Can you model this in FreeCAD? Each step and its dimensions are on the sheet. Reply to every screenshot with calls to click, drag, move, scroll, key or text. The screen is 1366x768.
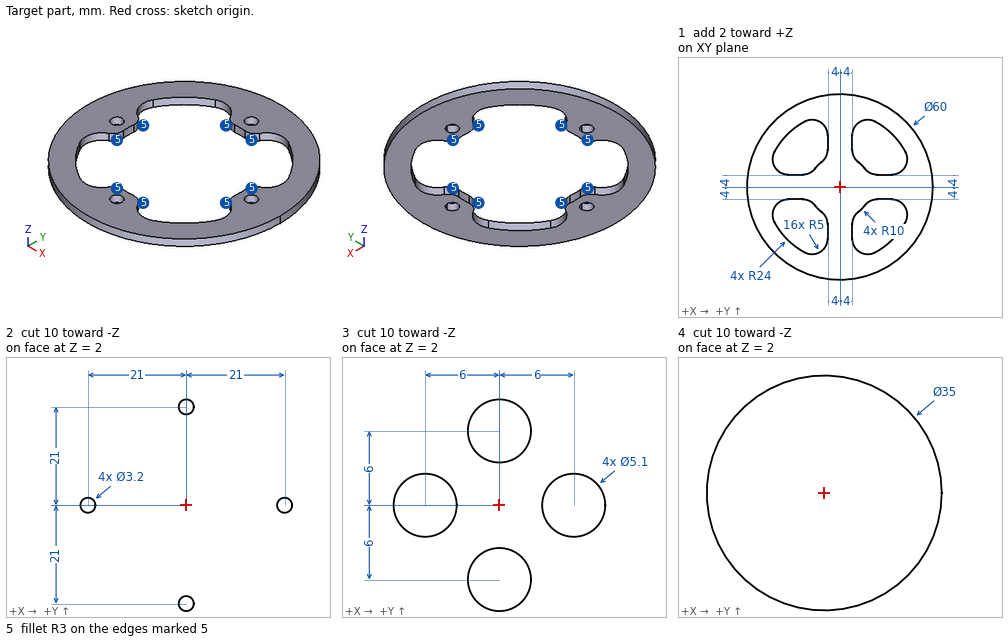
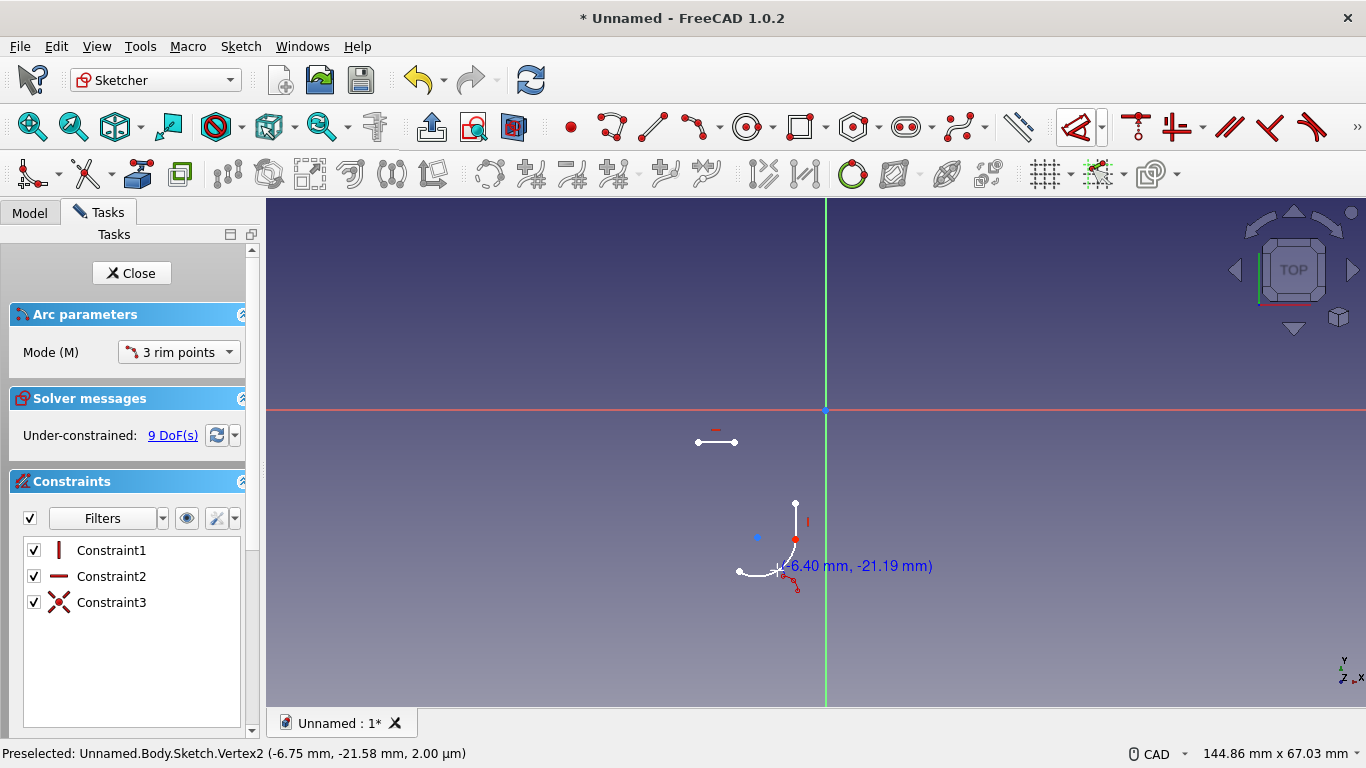
click(739, 572)
click(665, 496)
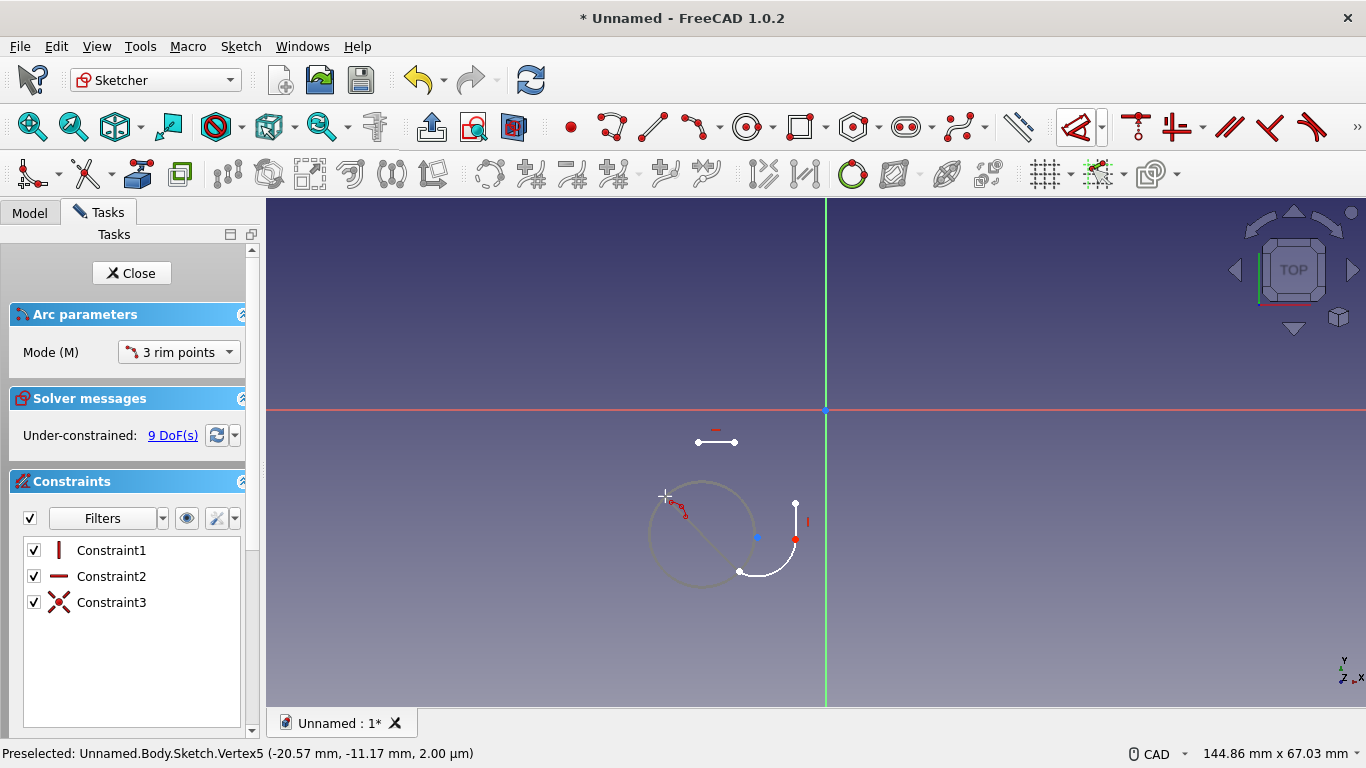
scroll(697, 539, up, 4)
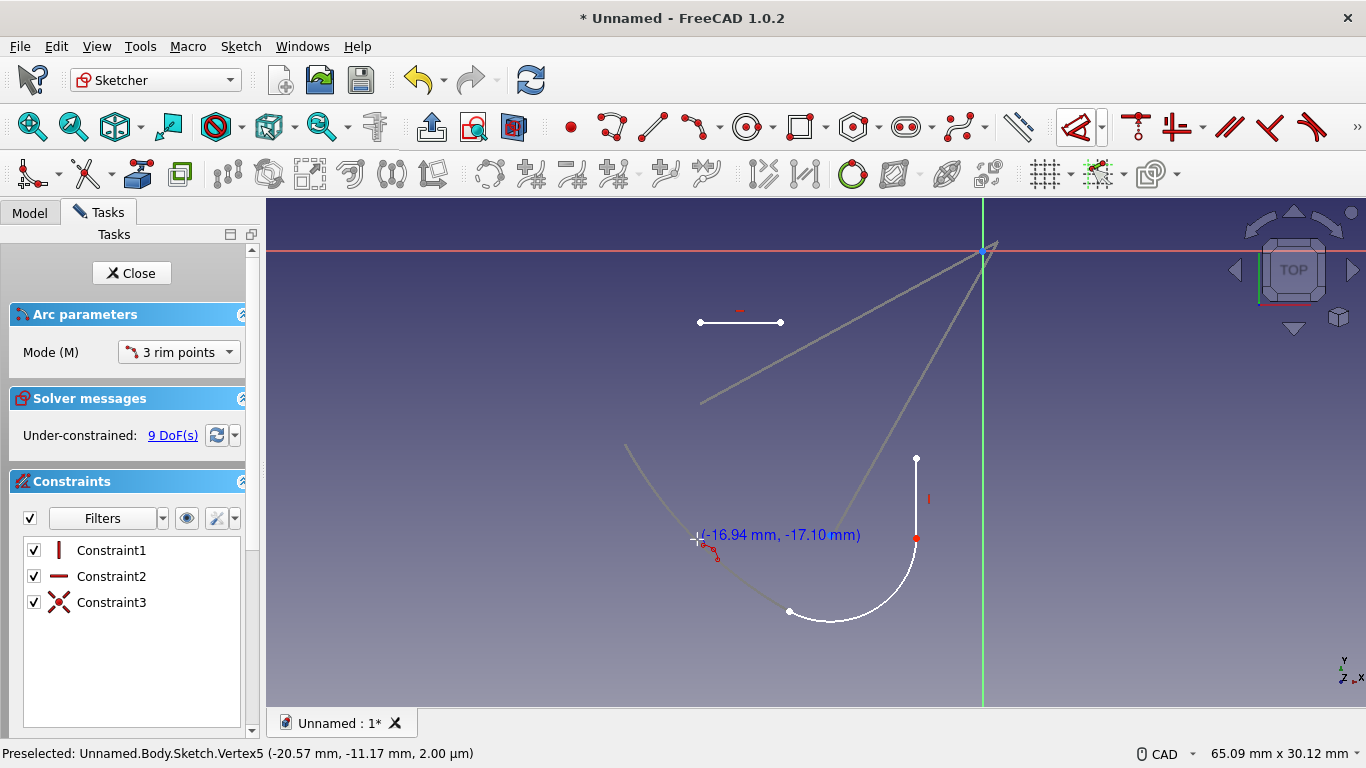
click(696, 538)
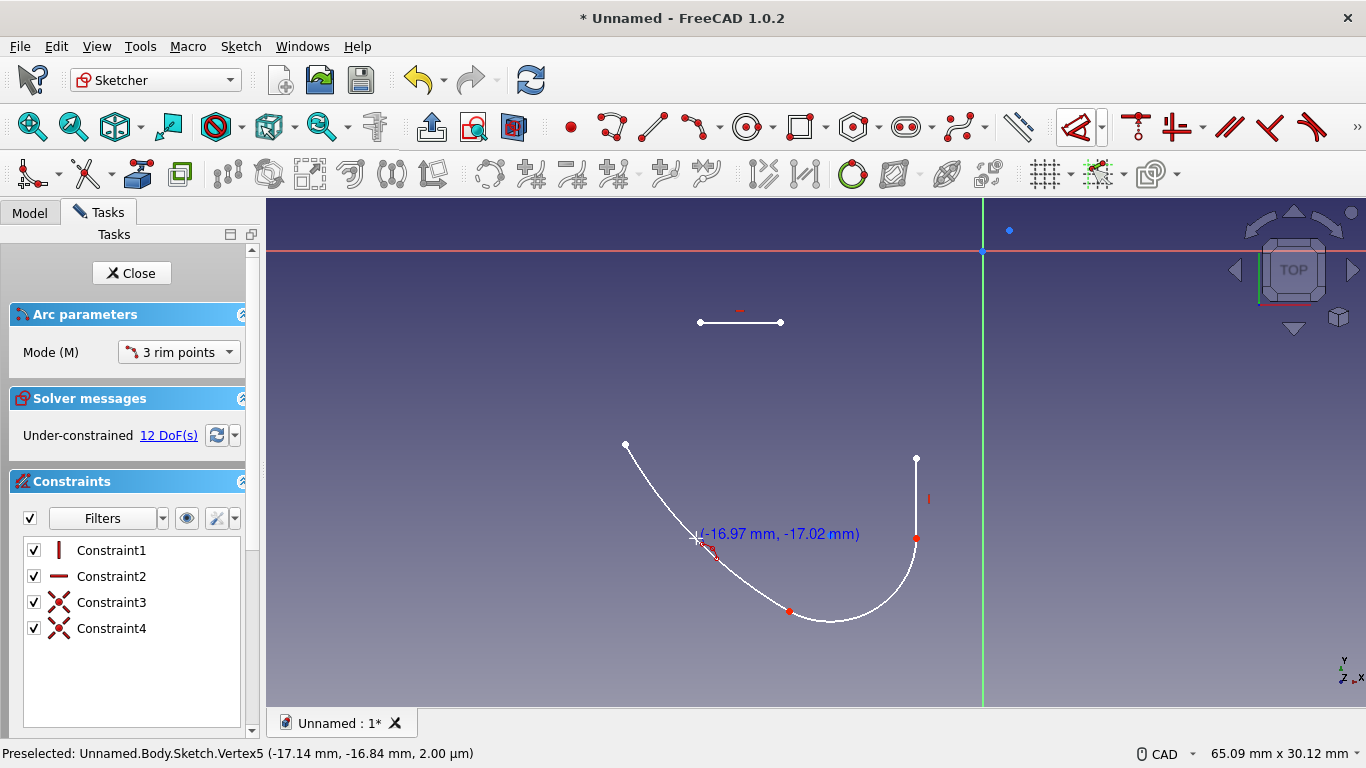
click(625, 445)
click(701, 323)
click(627, 360)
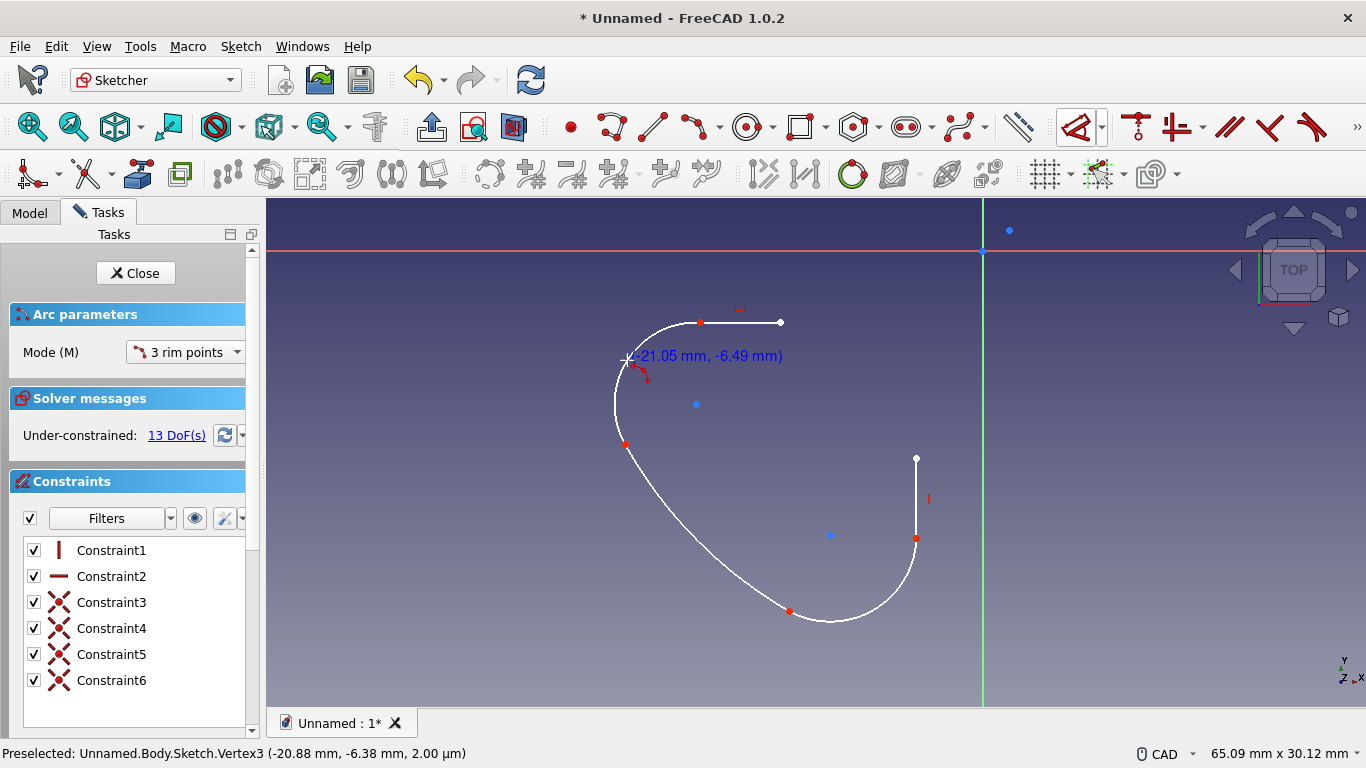
click(780, 323)
click(848, 353)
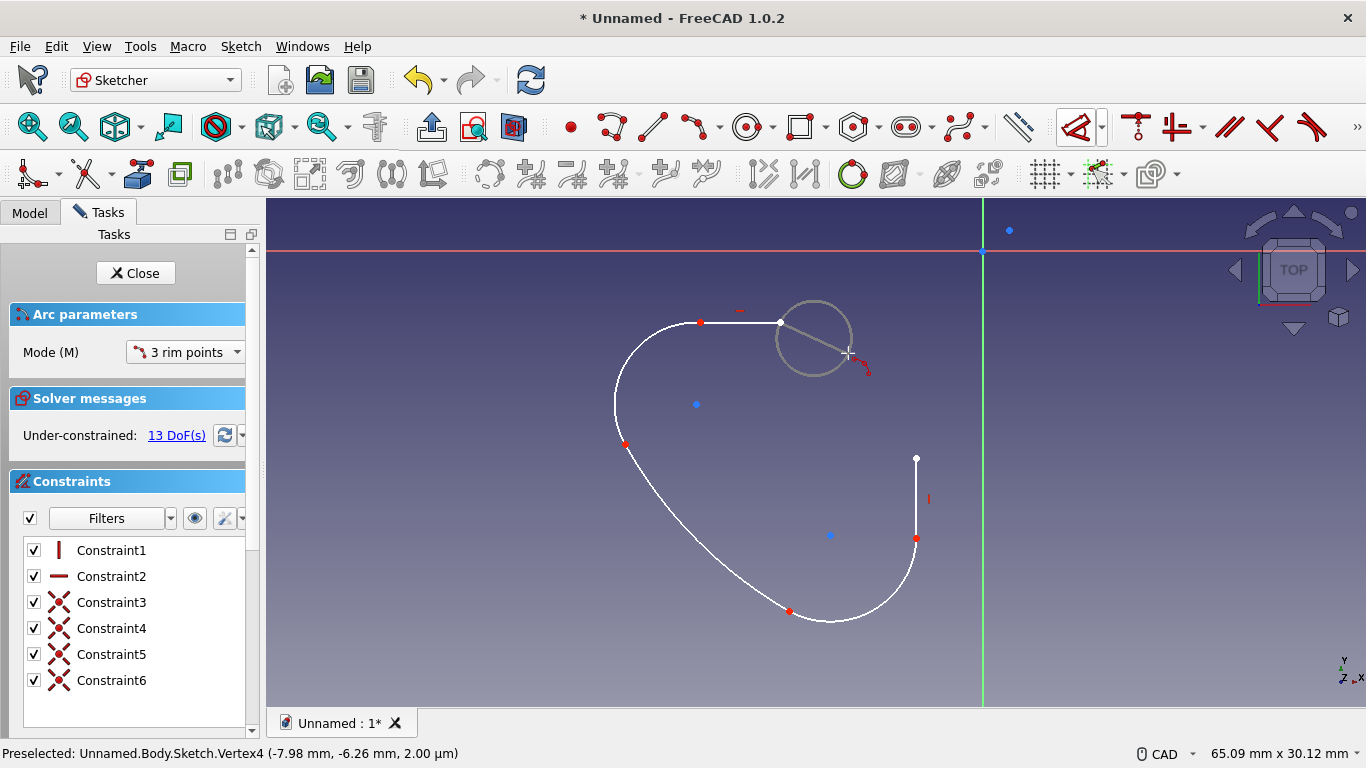
scroll(818, 328, up, 3)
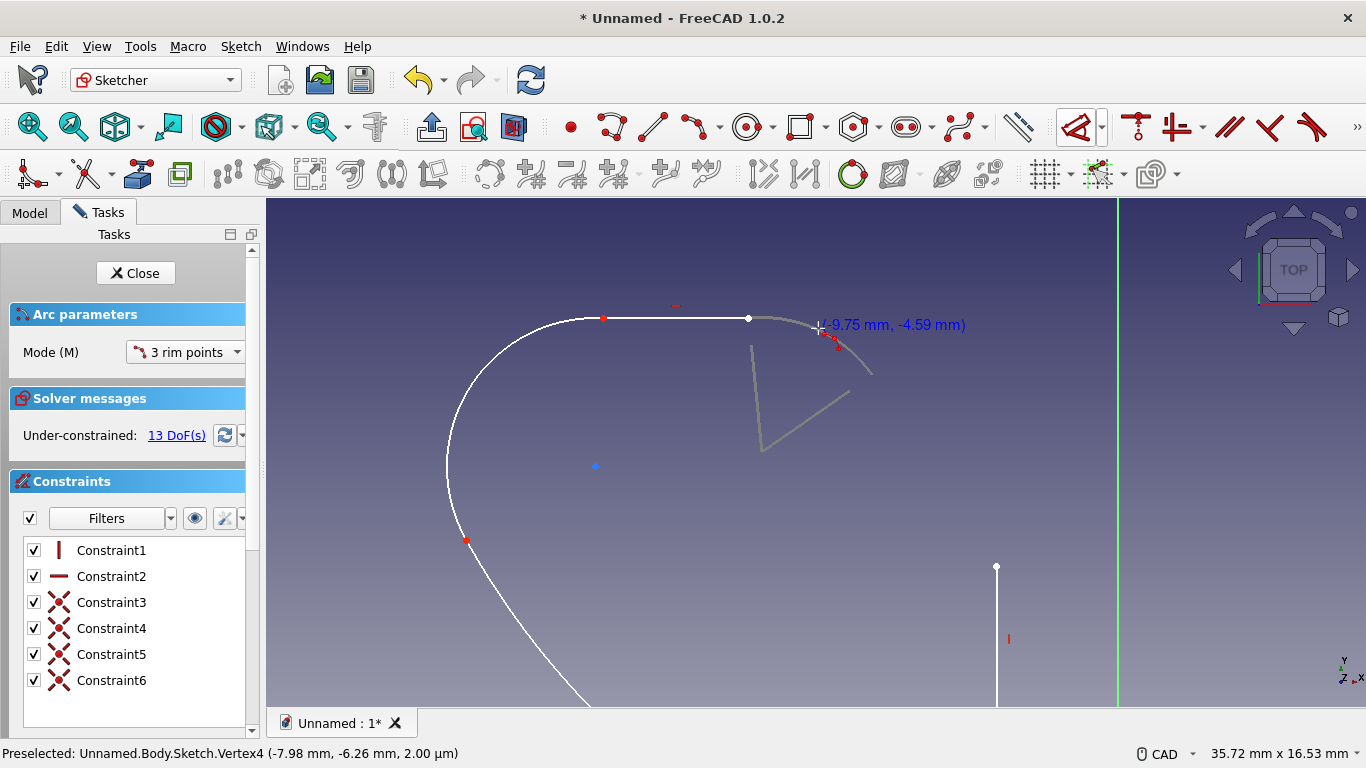
click(817, 328)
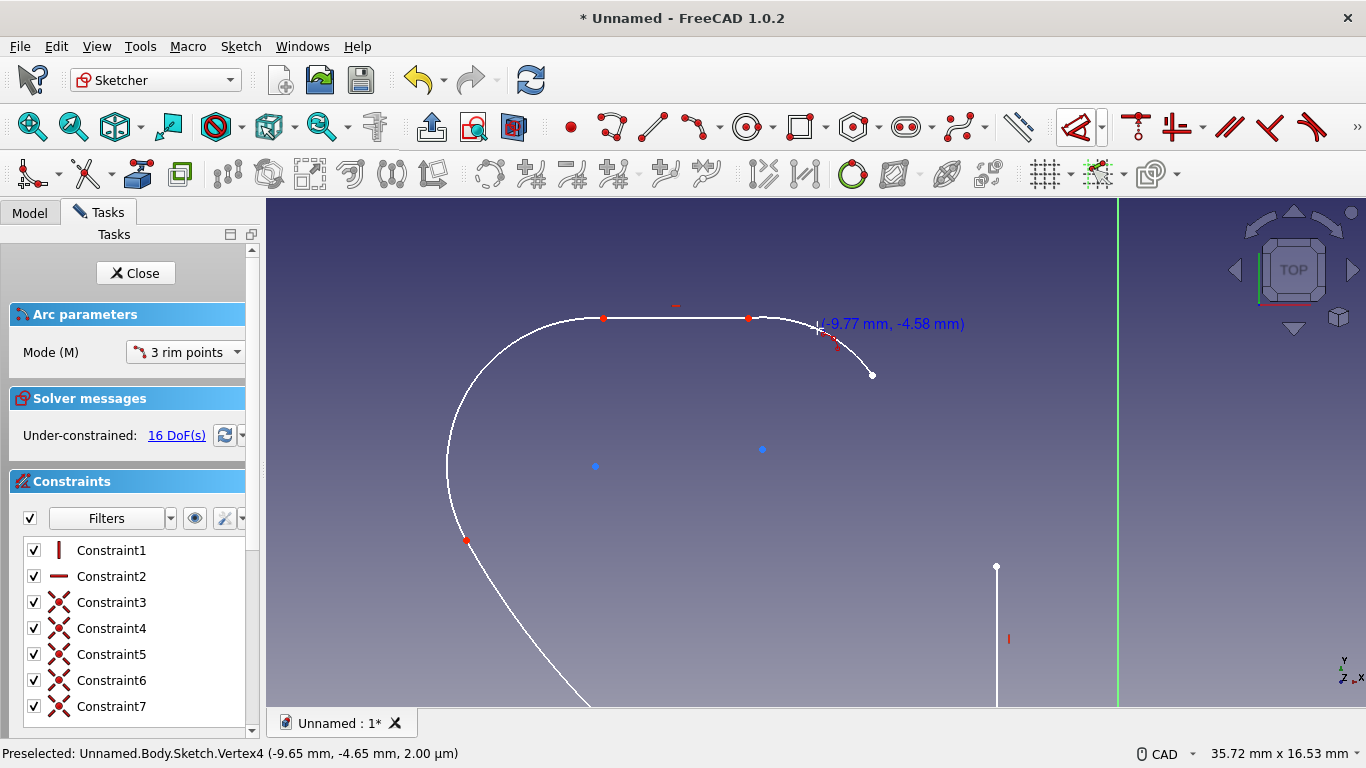
scroll(674, 505, down, 9)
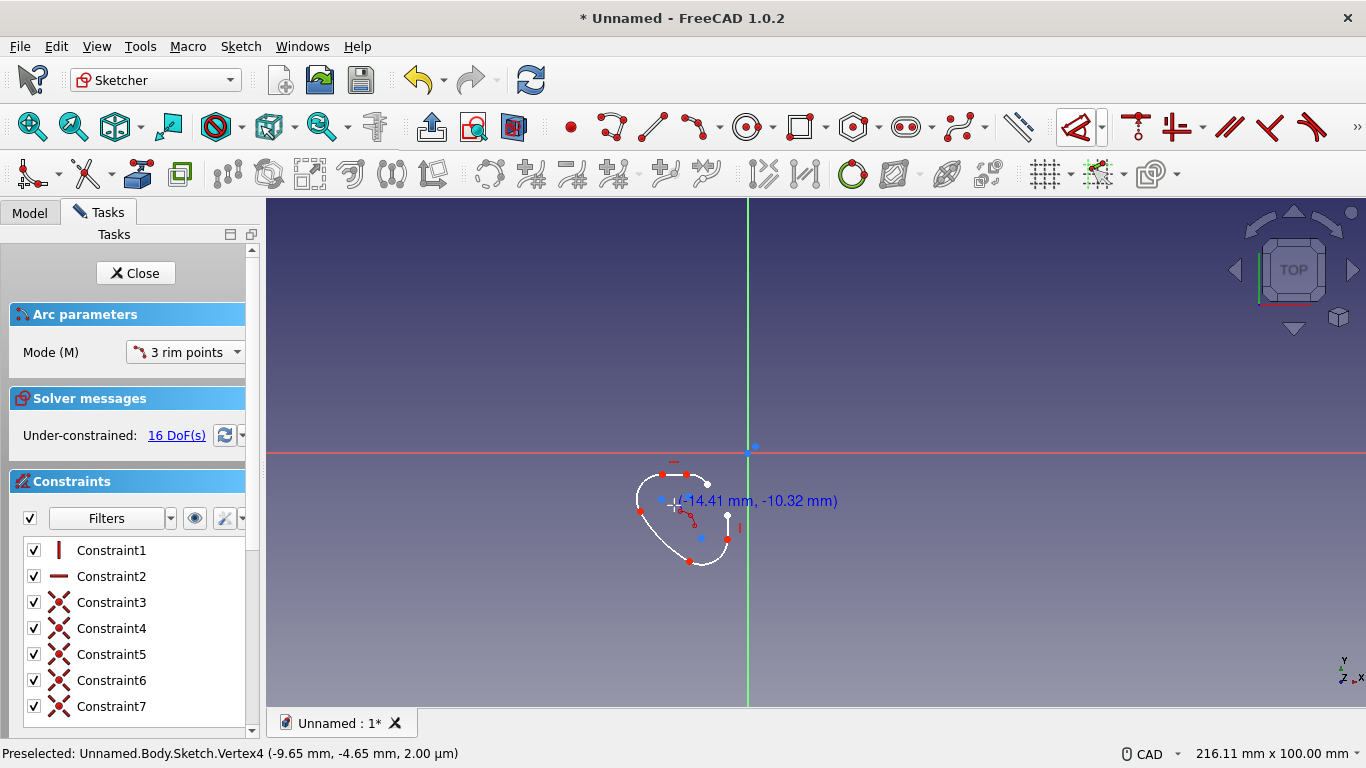
click(707, 484)
click(717, 494)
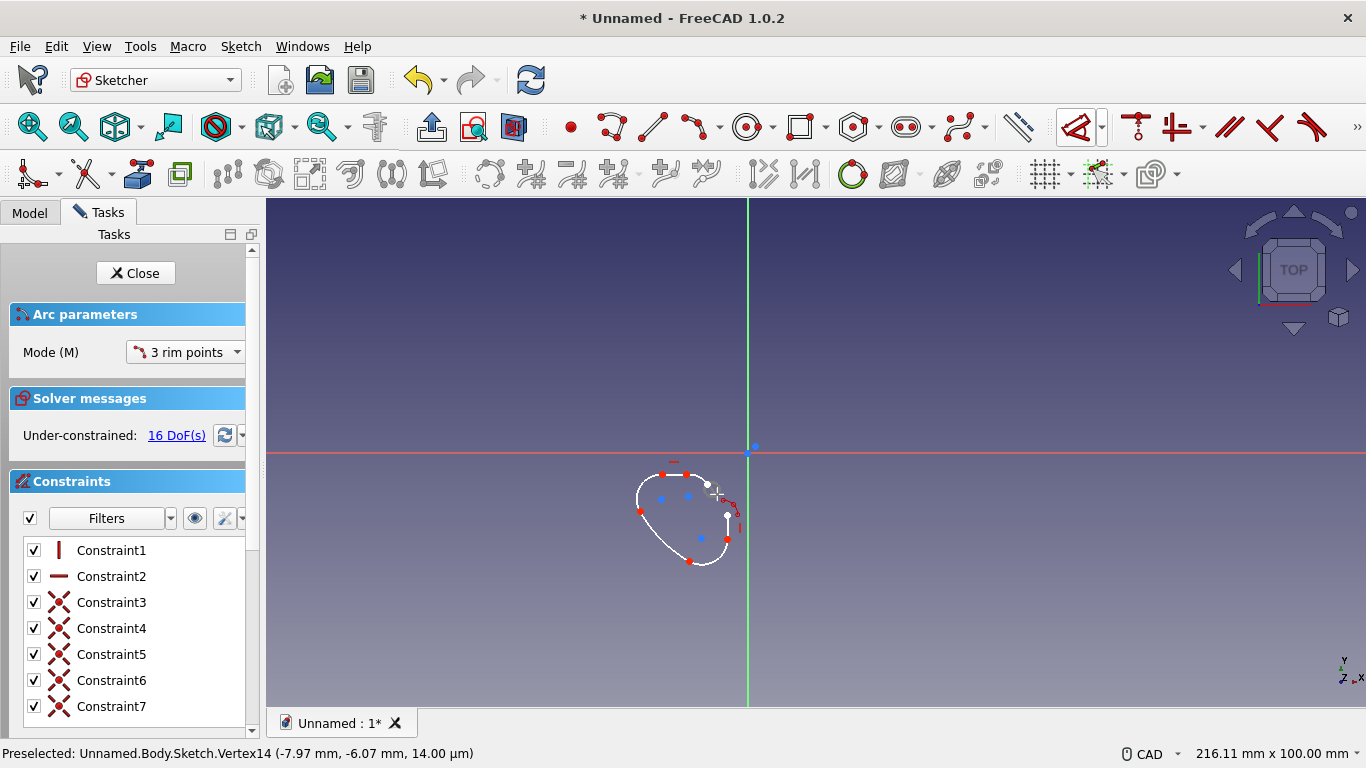
scroll(712, 489, up, 18)